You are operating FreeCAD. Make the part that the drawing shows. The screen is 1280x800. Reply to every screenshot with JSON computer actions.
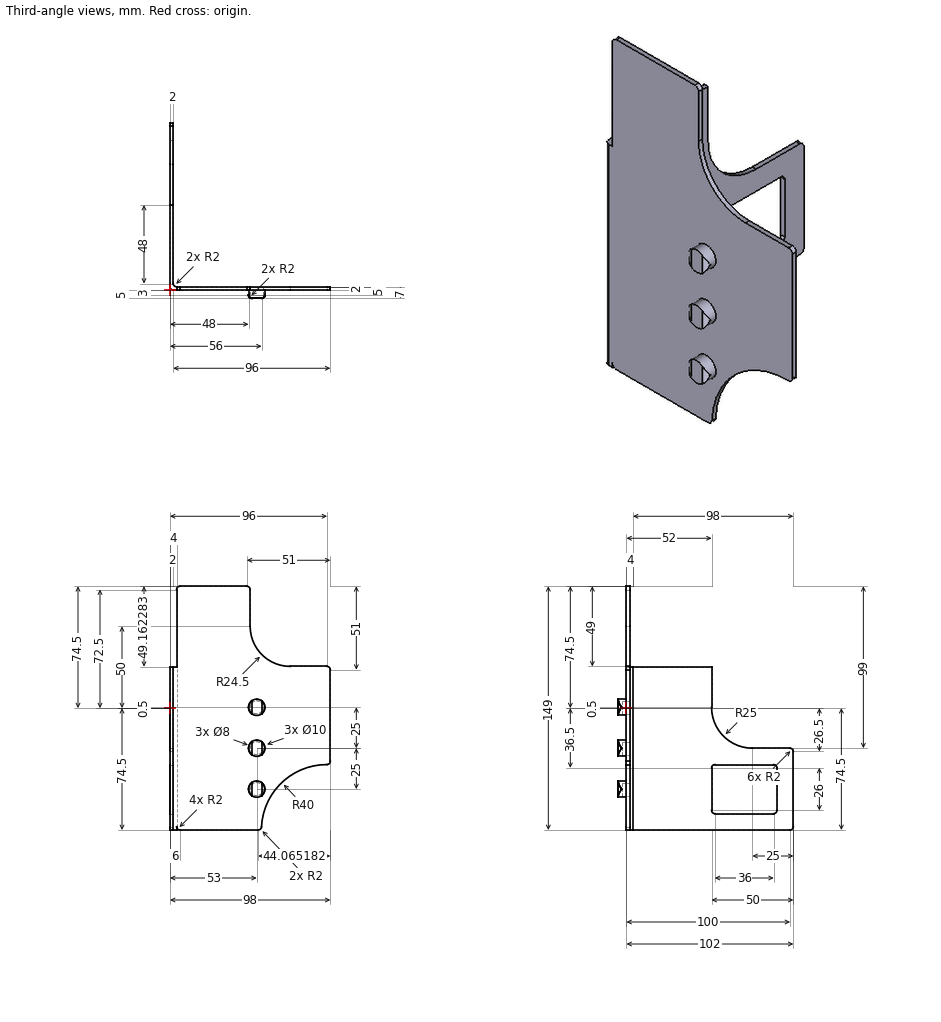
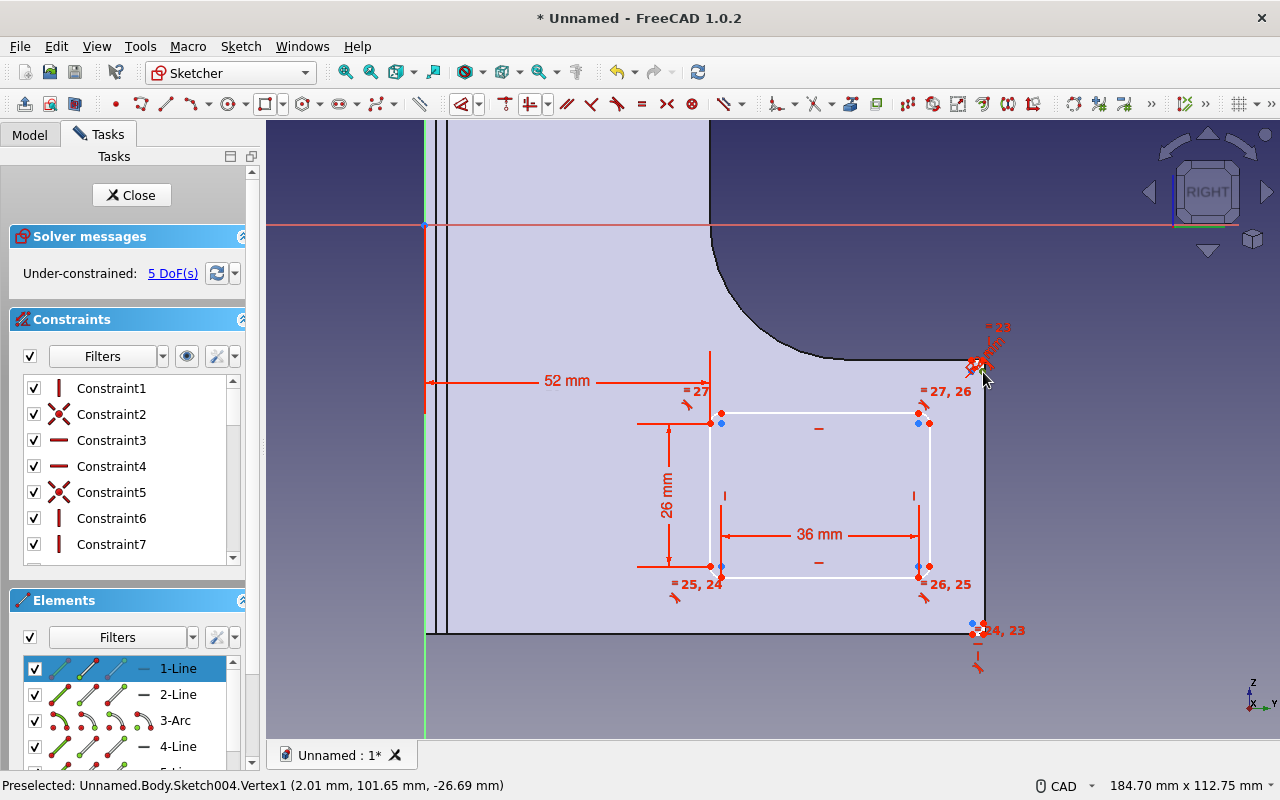
{"action": "key", "text": "l"}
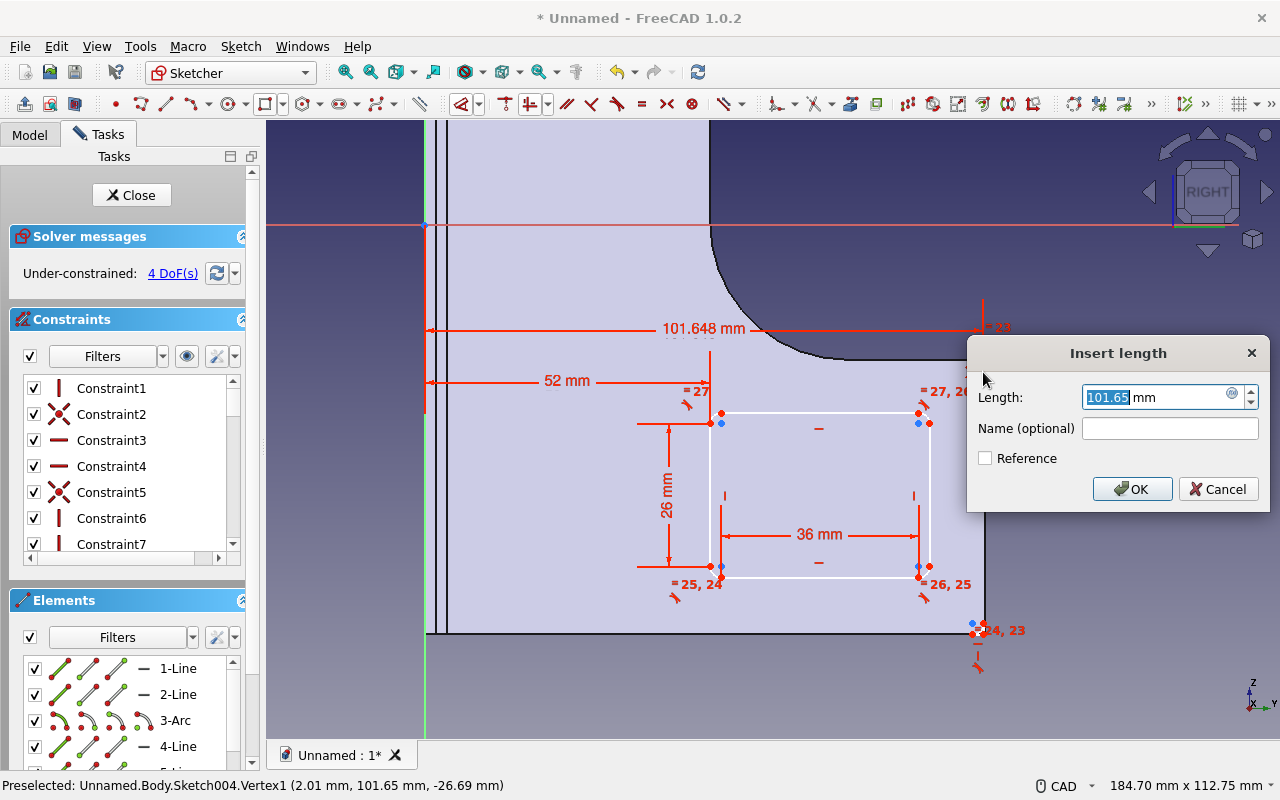
{"action": "type", "text": "102"}
{"action": "key", "text": "Return"}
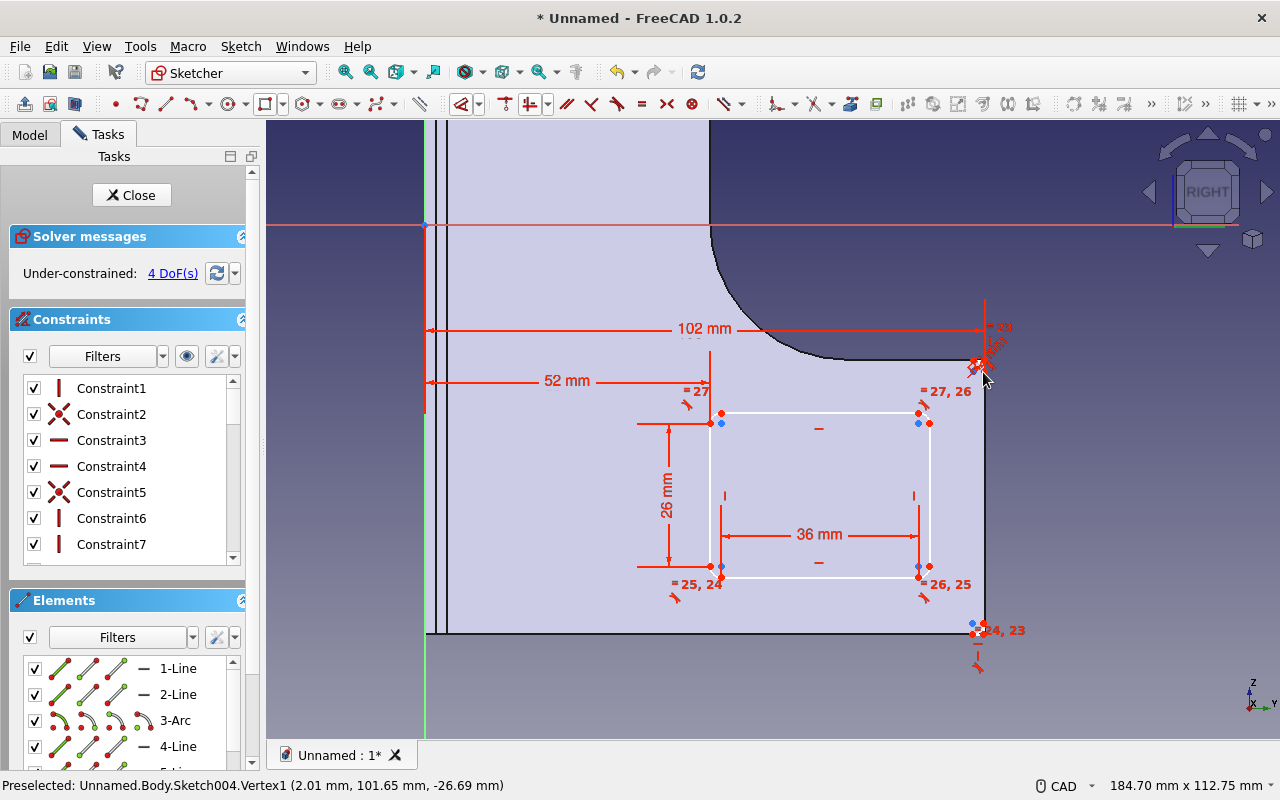
{"action": "left_click", "coordinate": [973, 635]}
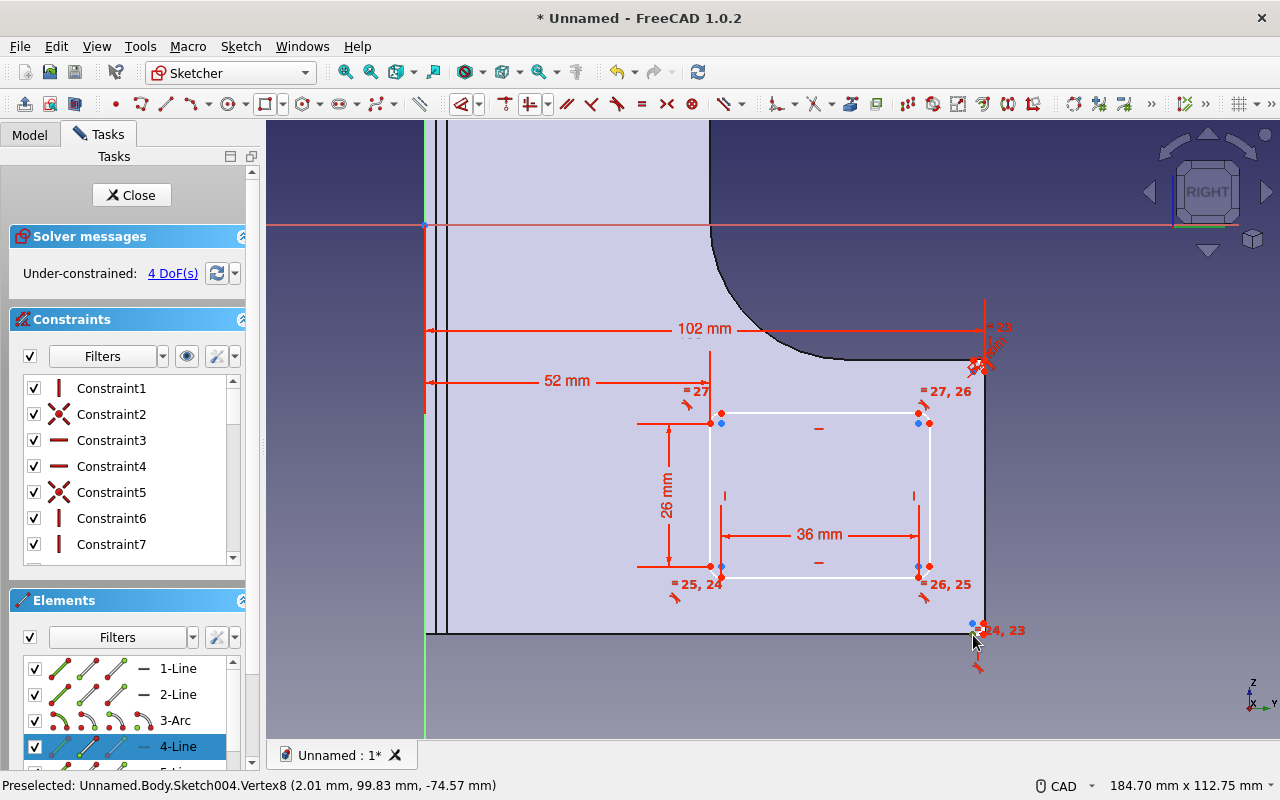
{"action": "key", "text": "l"}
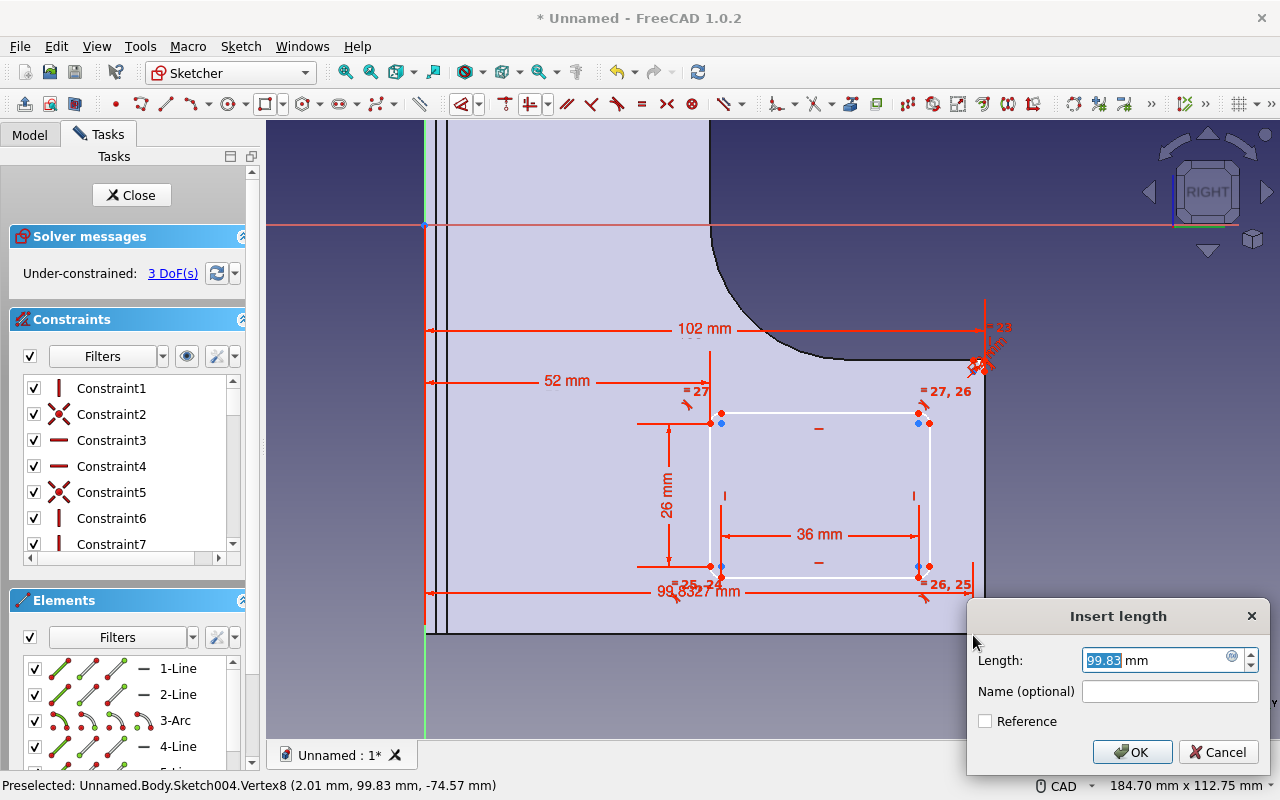
{"action": "type", "text": "100"}
{"action": "key", "text": "Return"}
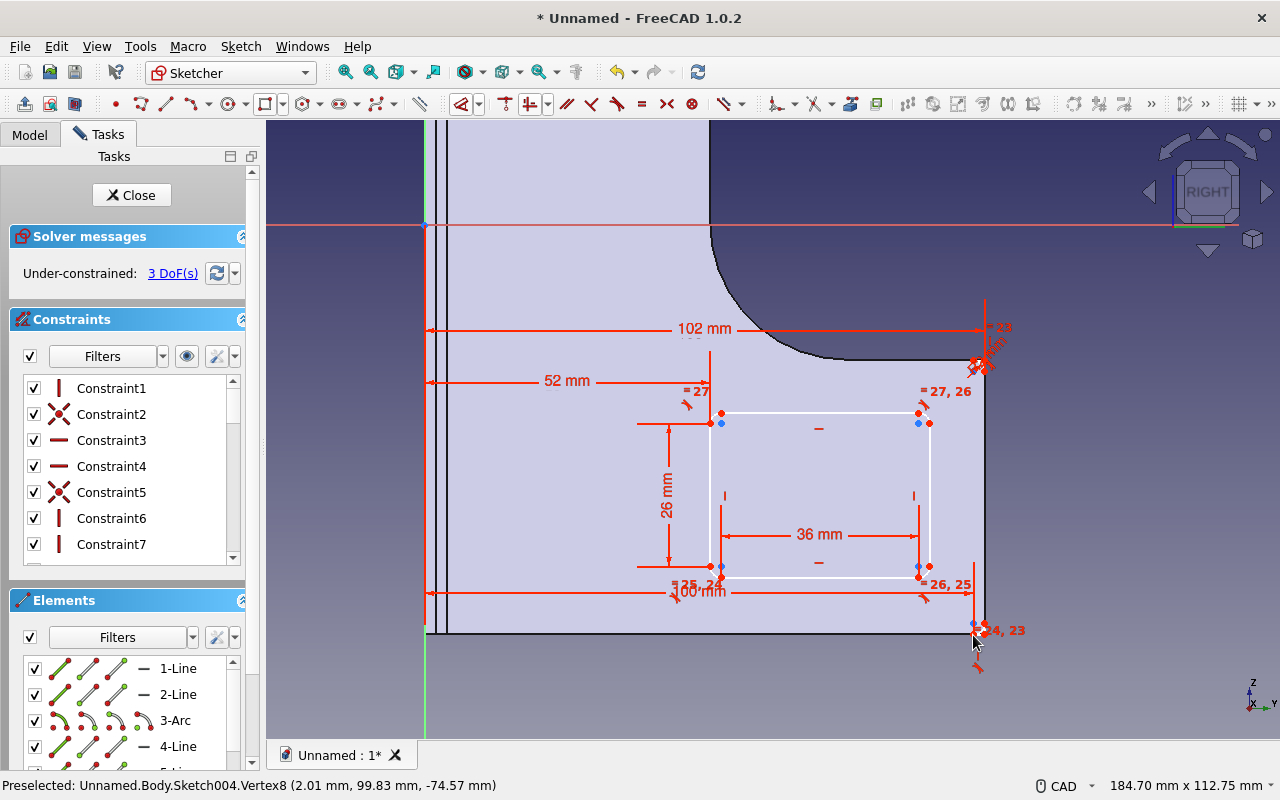
{"action": "left_click", "coordinate": [985, 372]}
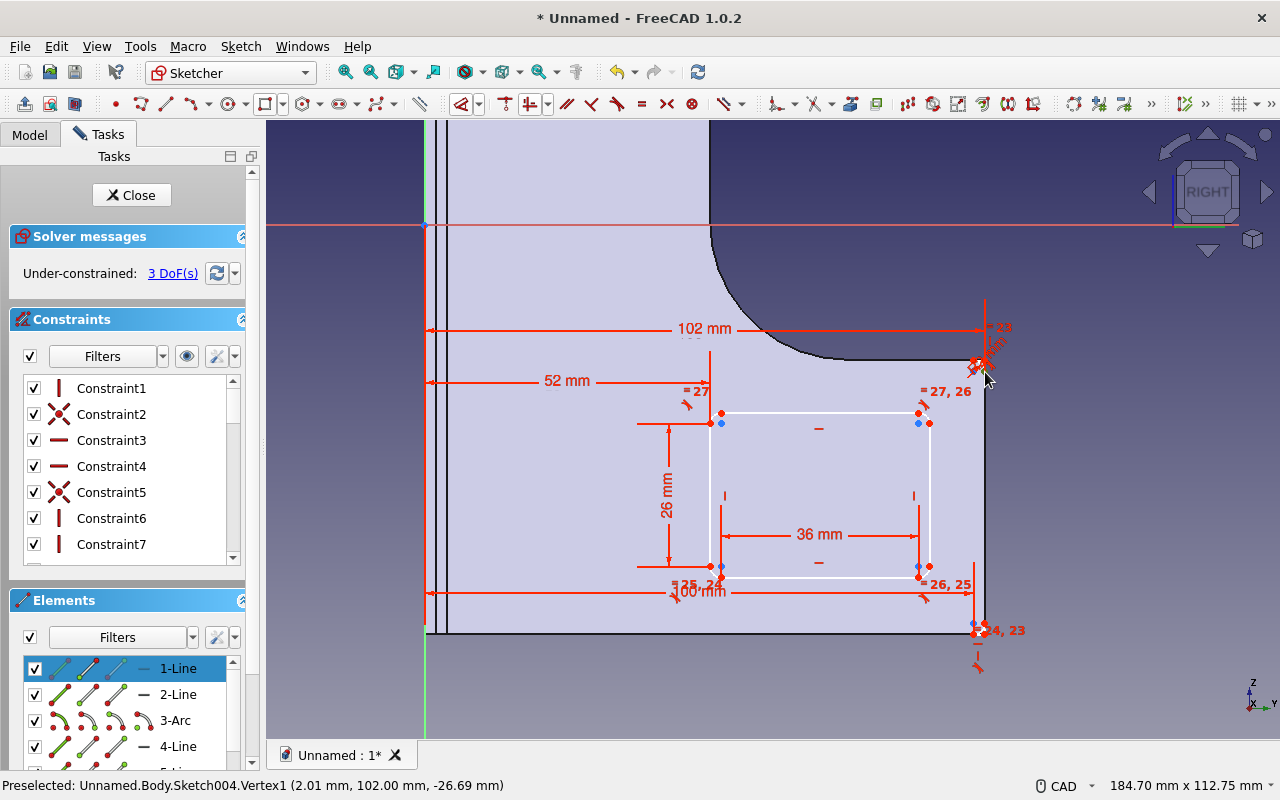
{"action": "key", "text": "i"}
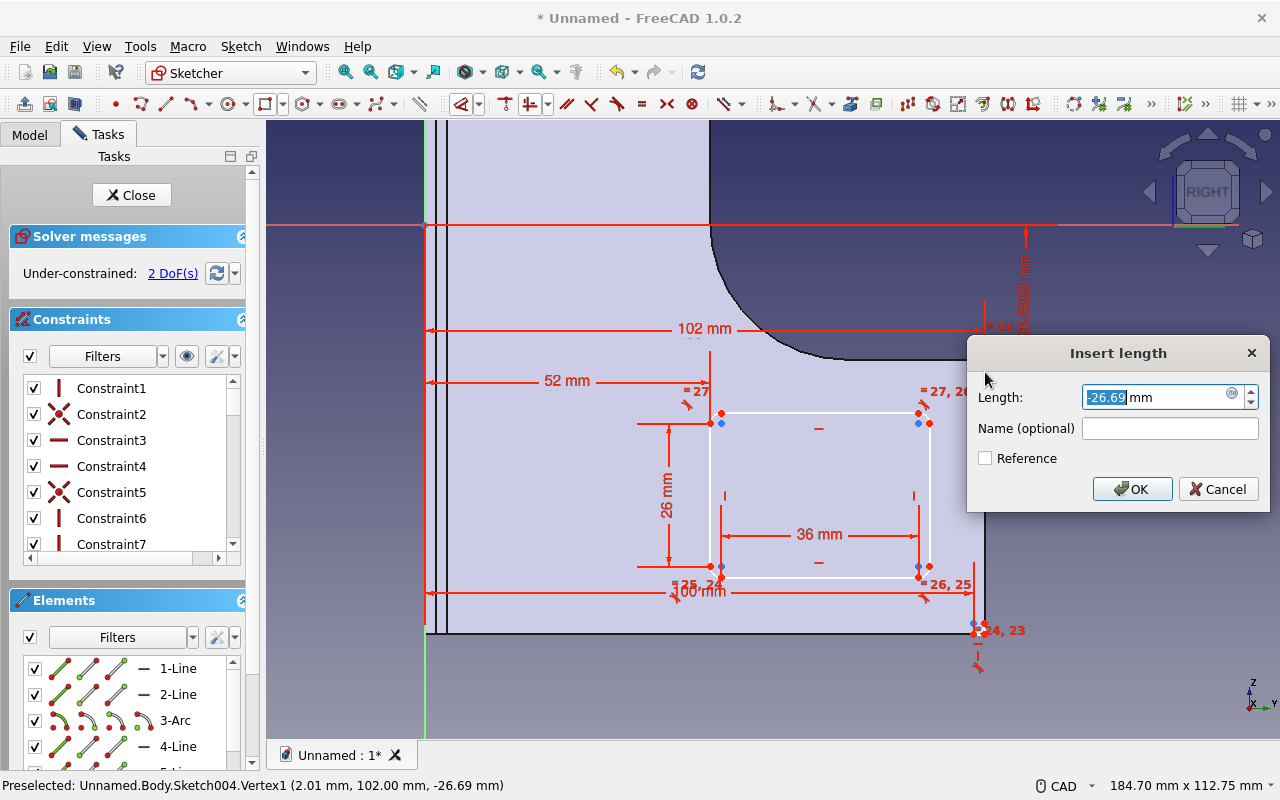
{"action": "type", "text": "-26.5"}
{"action": "key", "text": "Return"}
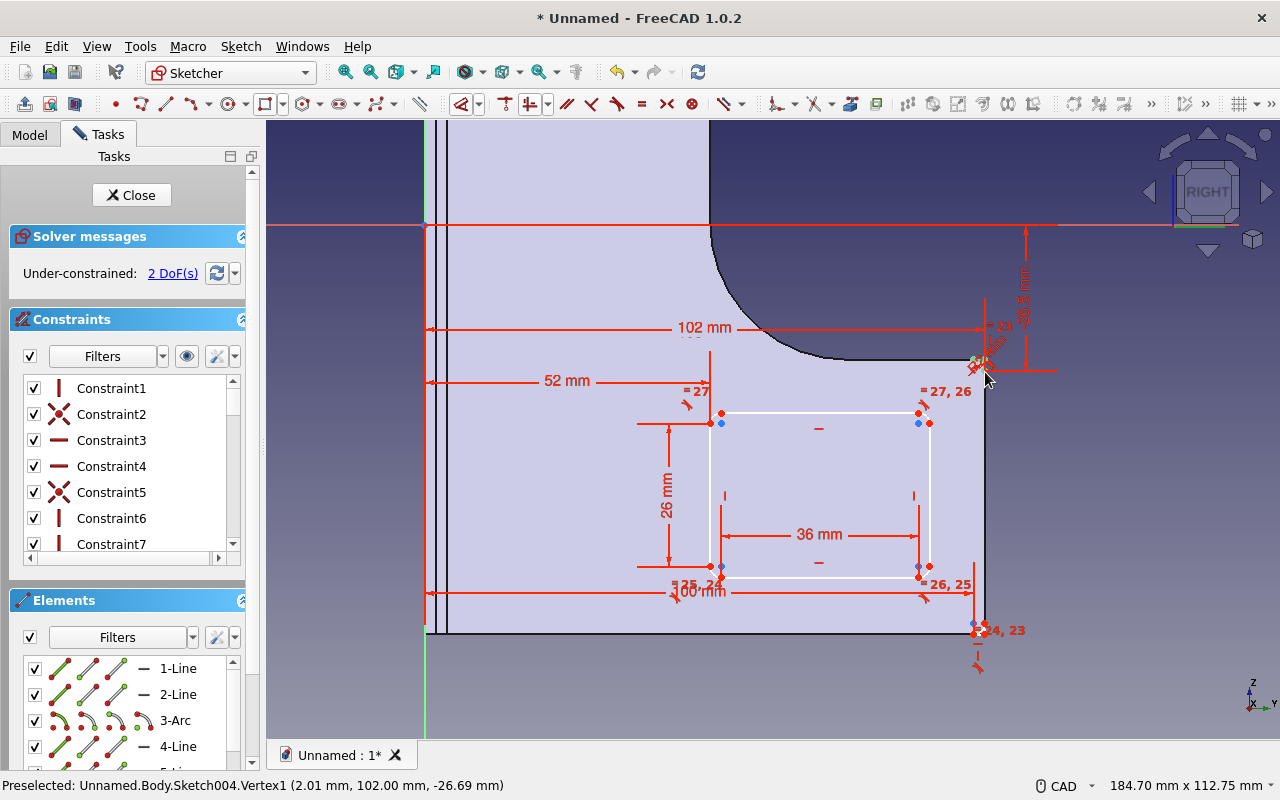
{"action": "left_click", "coordinate": [974, 635]}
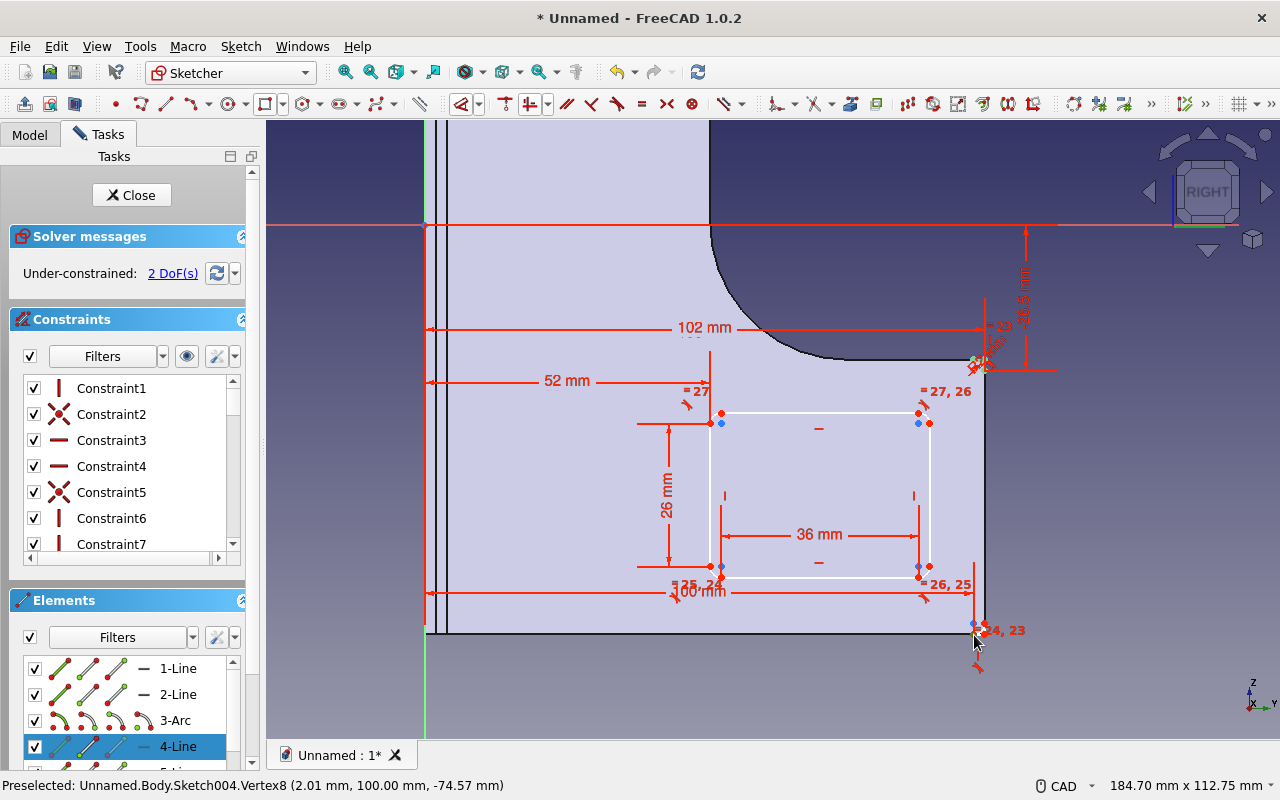
{"action": "left_click", "coordinate": [478, 104]}